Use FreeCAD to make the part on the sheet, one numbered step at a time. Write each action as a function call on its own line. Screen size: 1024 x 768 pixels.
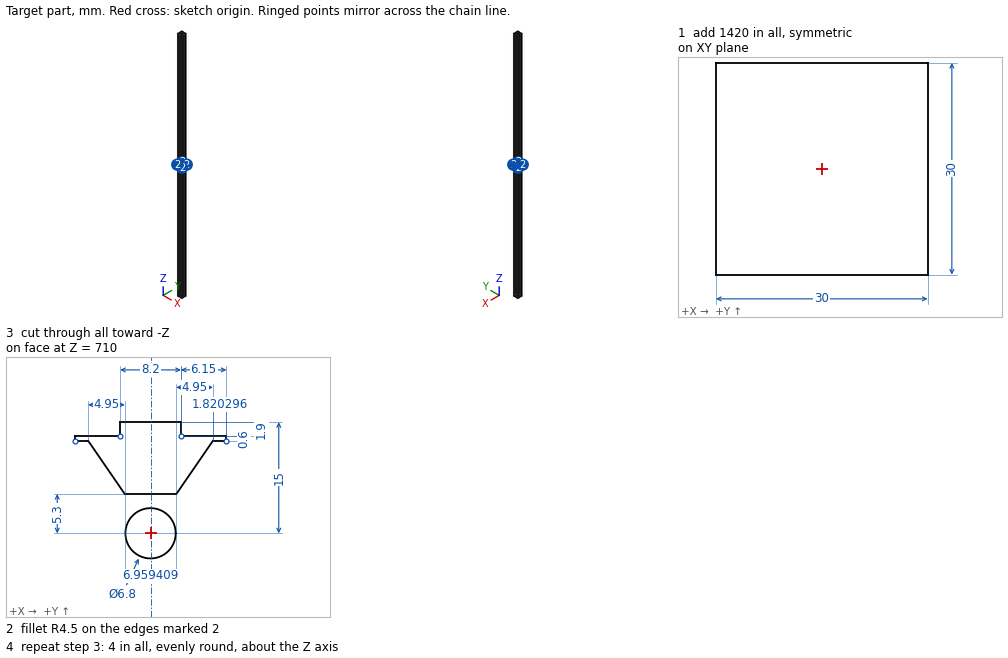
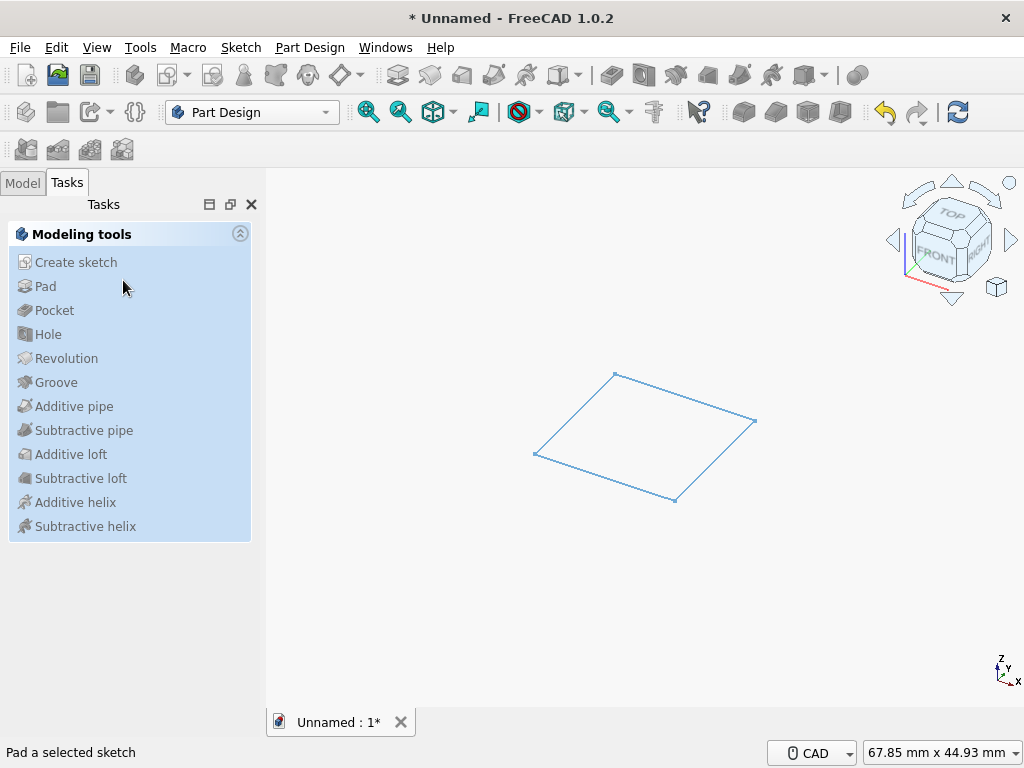
click(398, 76)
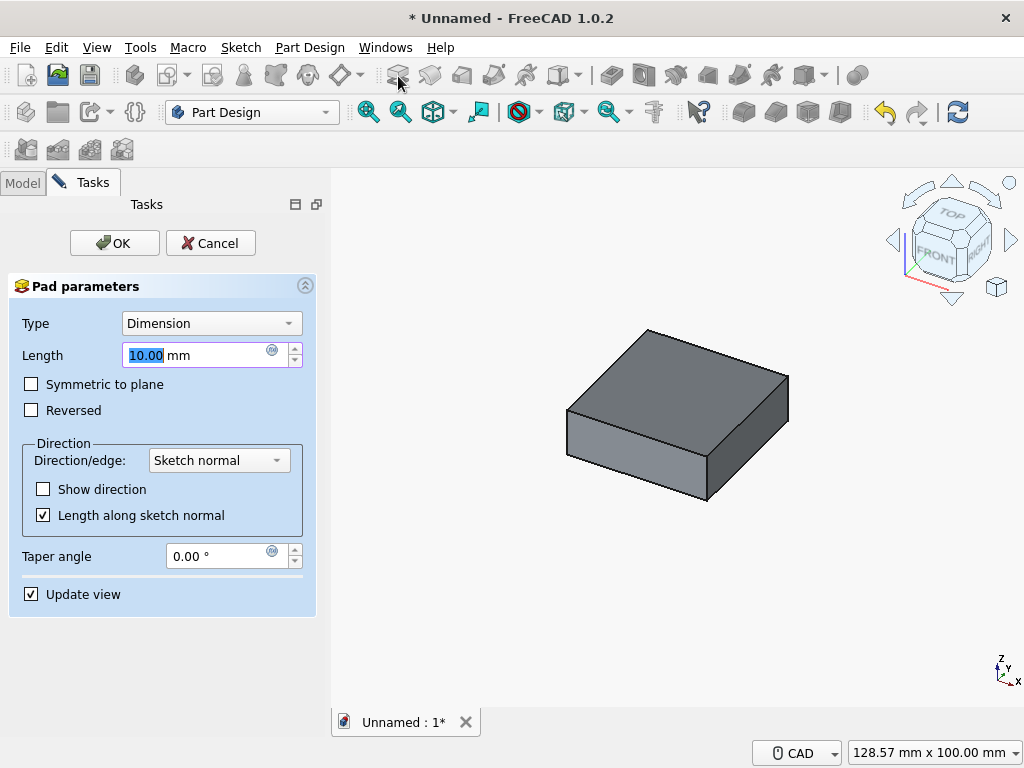
text(1420)
key(Tab)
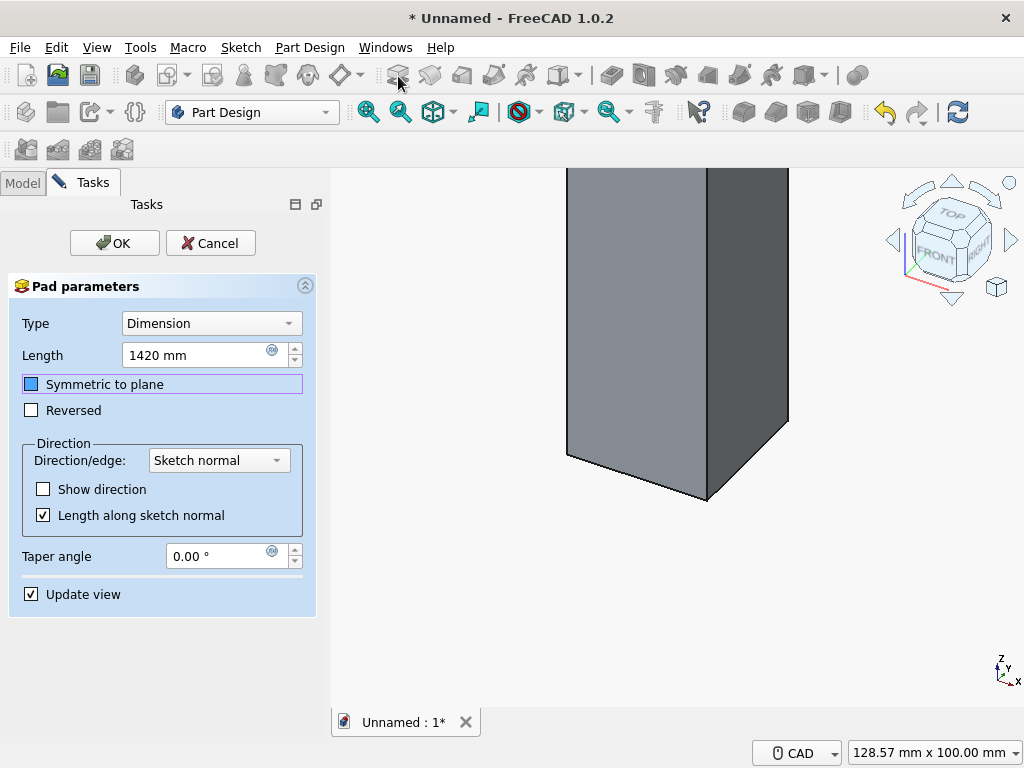
click(30, 384)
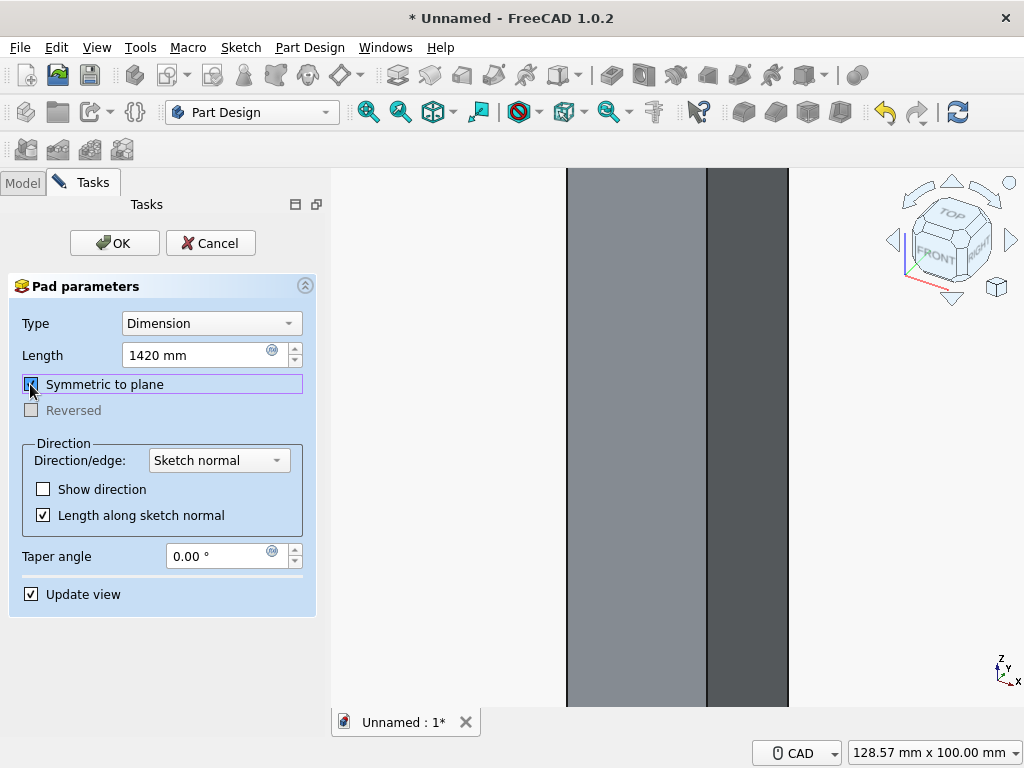
click(115, 243)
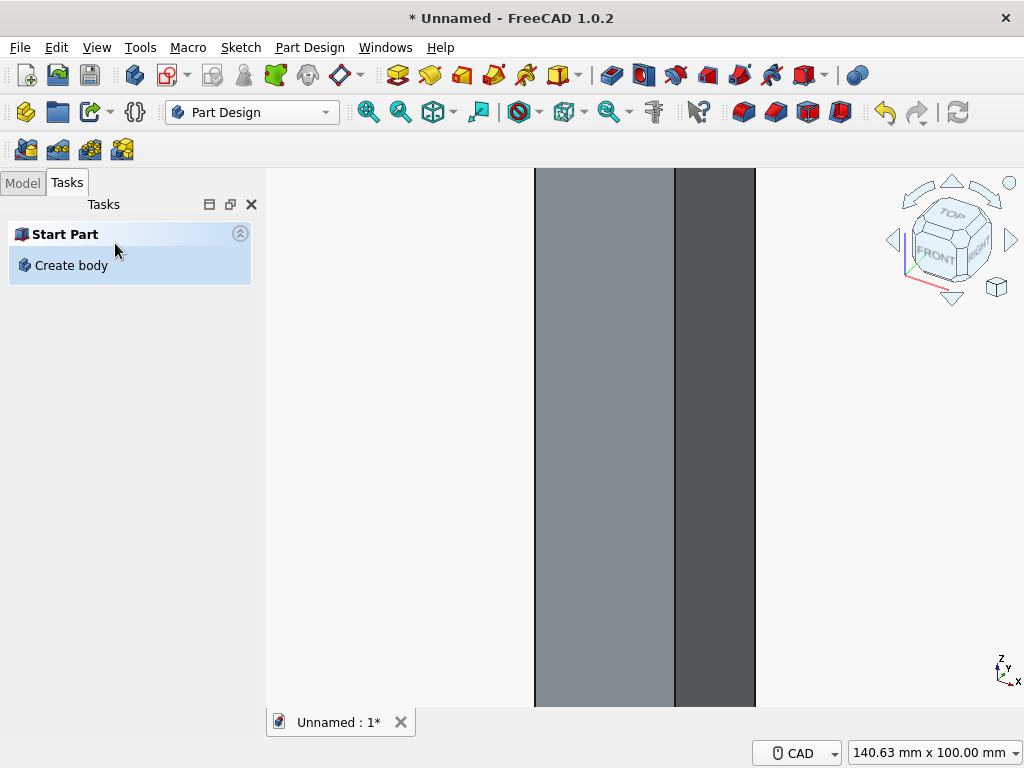
click(370, 112)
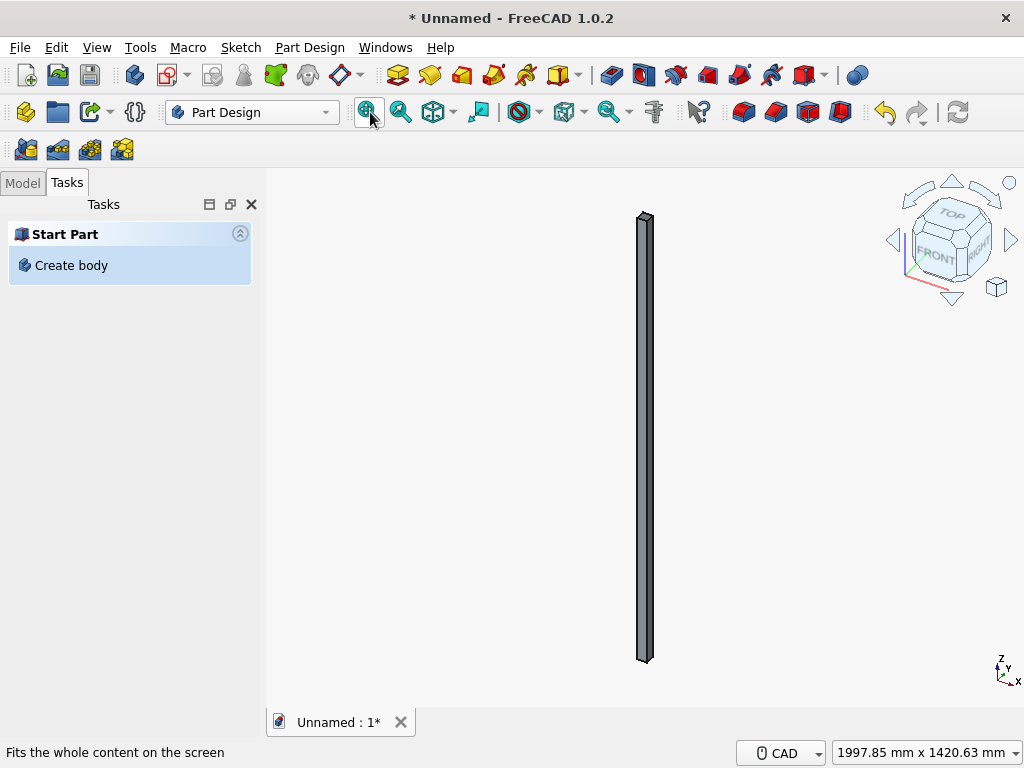
click(647, 441)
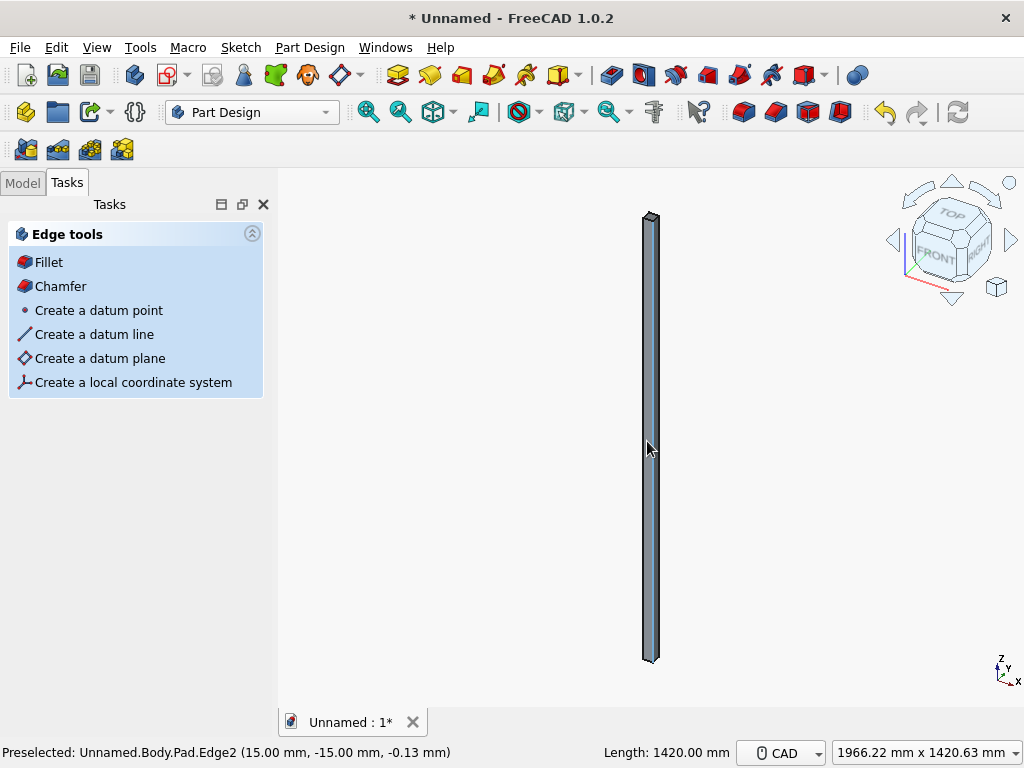
key(0)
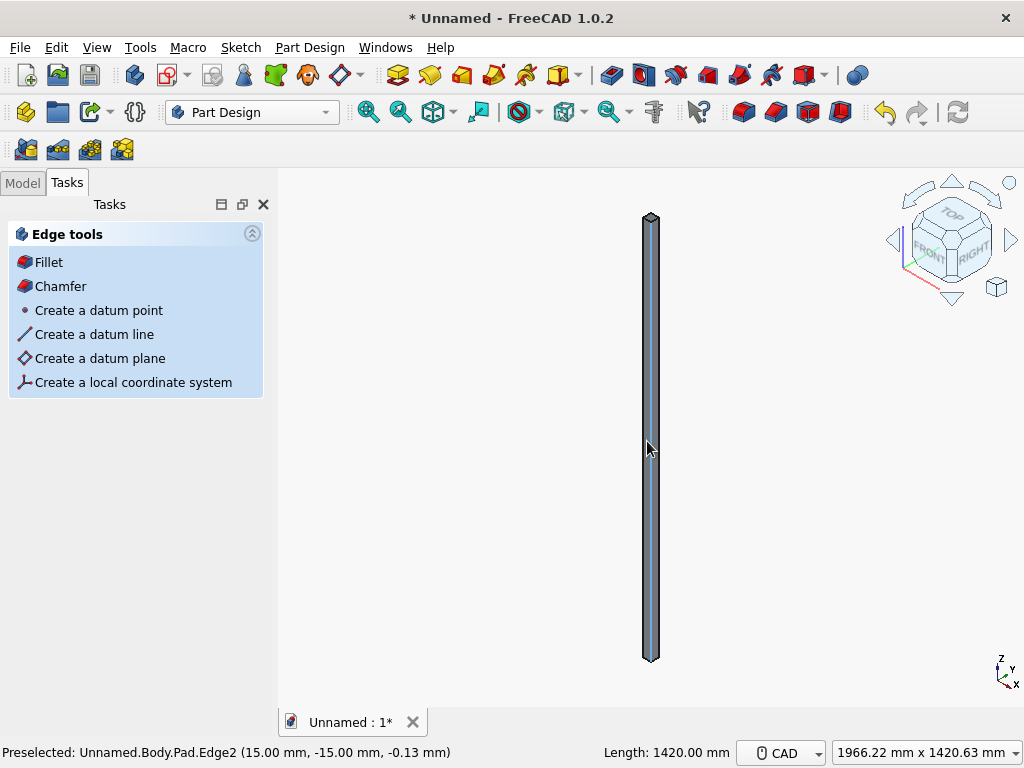
key(2)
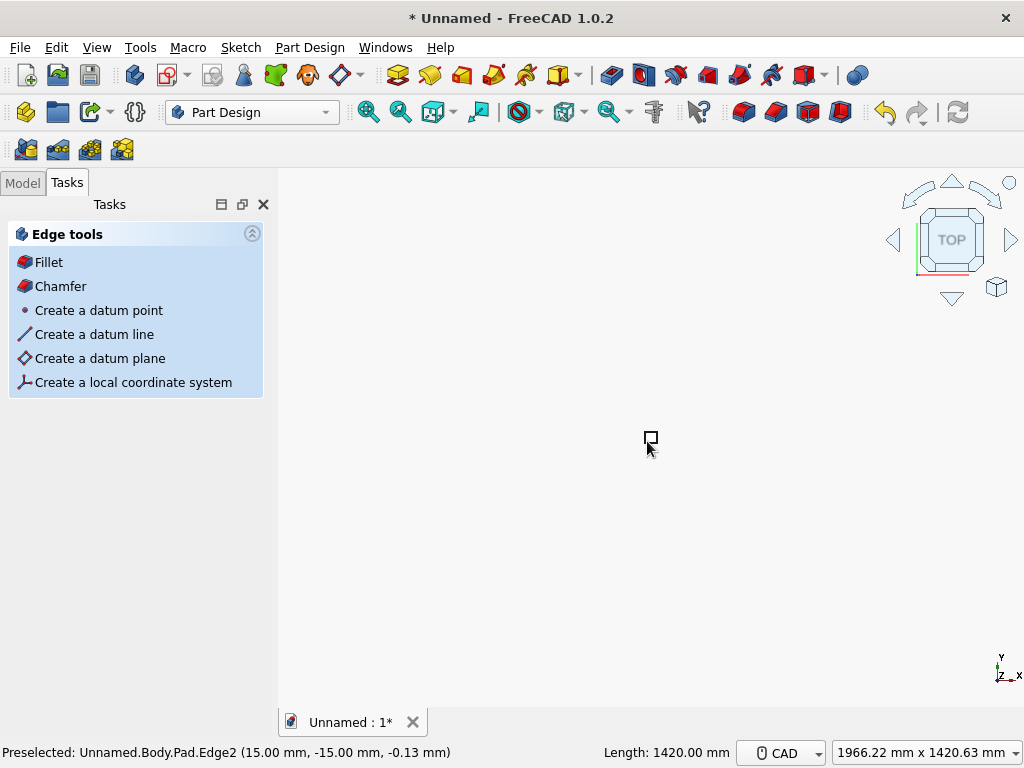
key(v)
key(f)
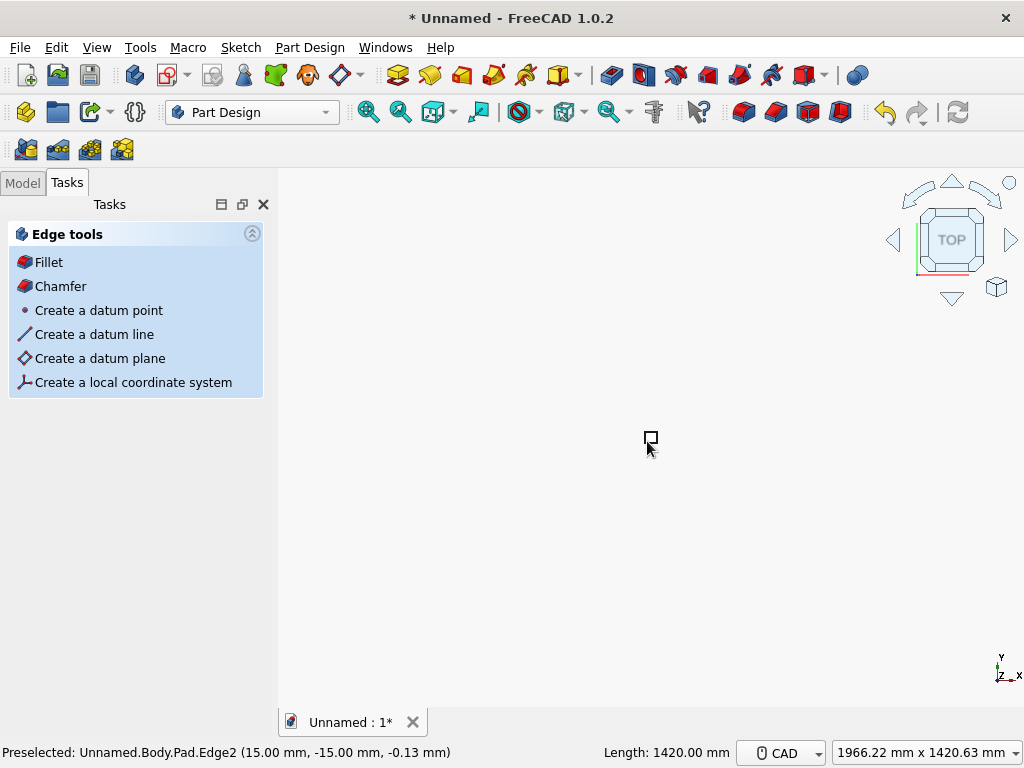
key(1)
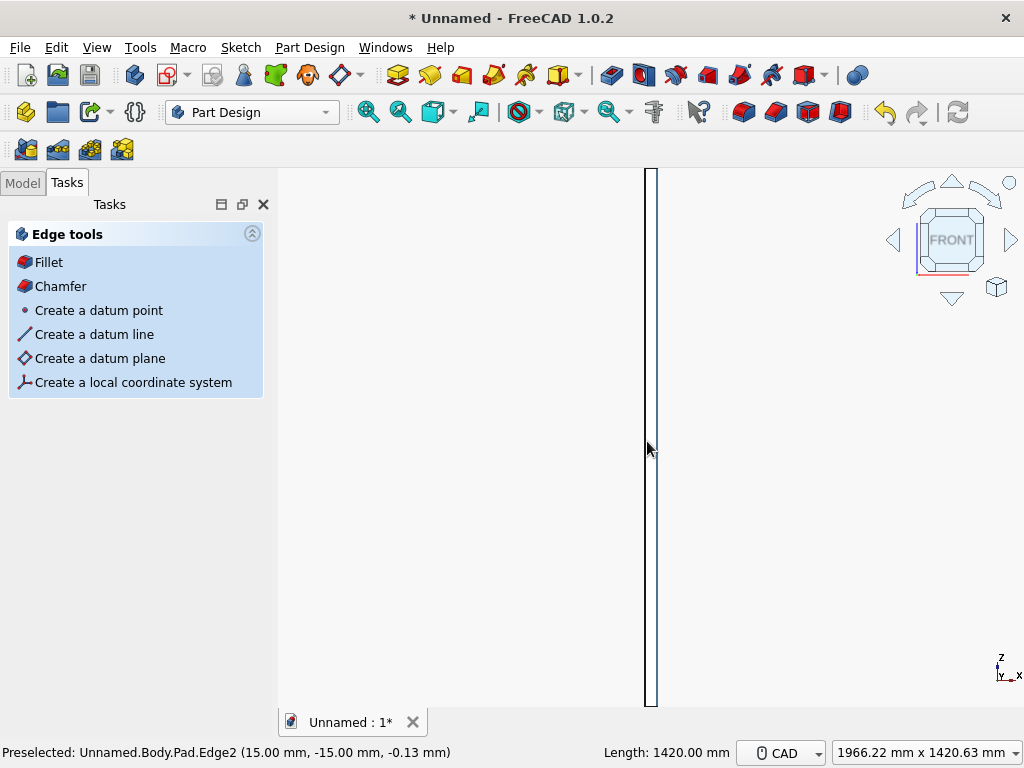
key(v)
key(f)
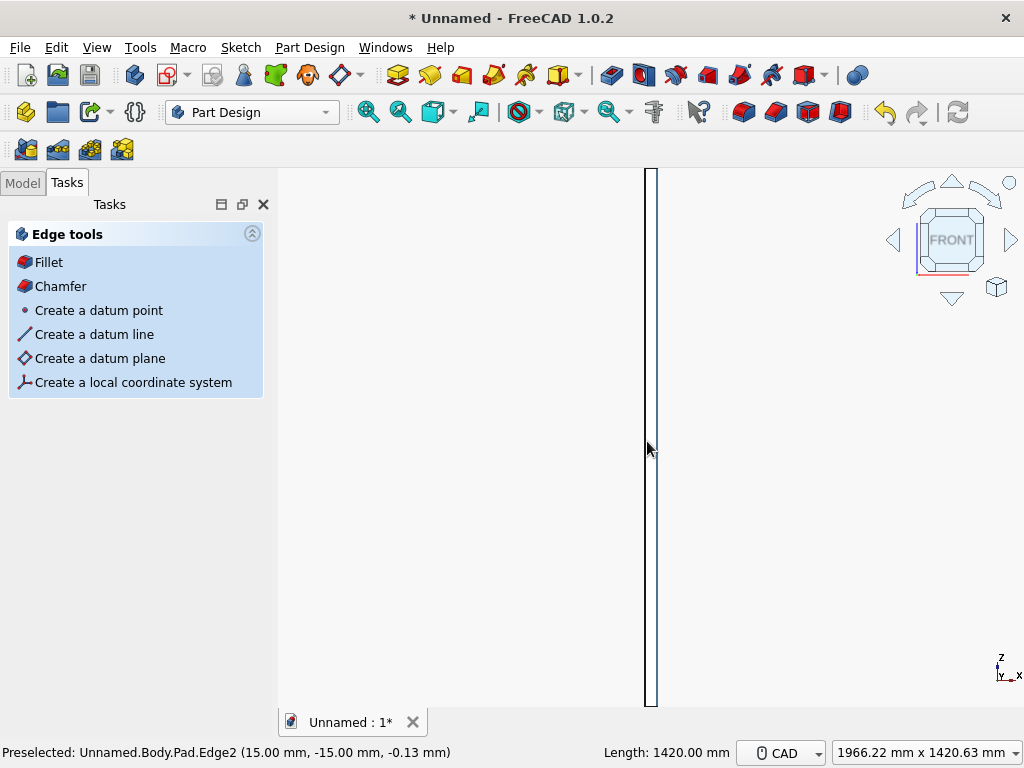
click(645, 437, ctrl)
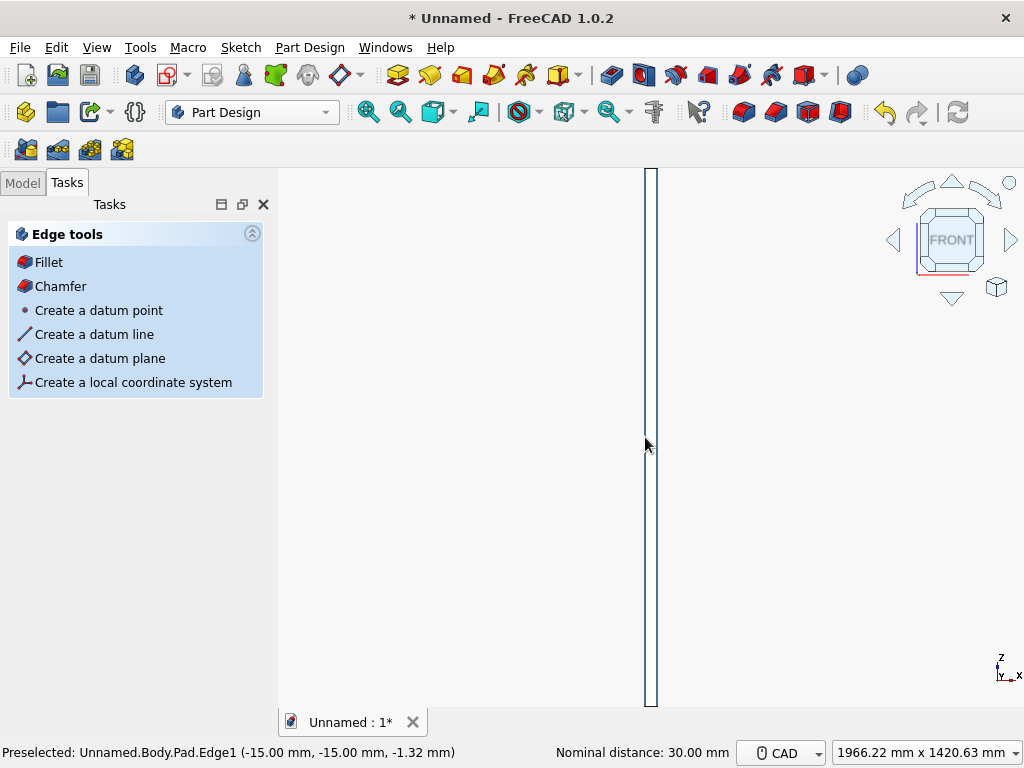
key(3)